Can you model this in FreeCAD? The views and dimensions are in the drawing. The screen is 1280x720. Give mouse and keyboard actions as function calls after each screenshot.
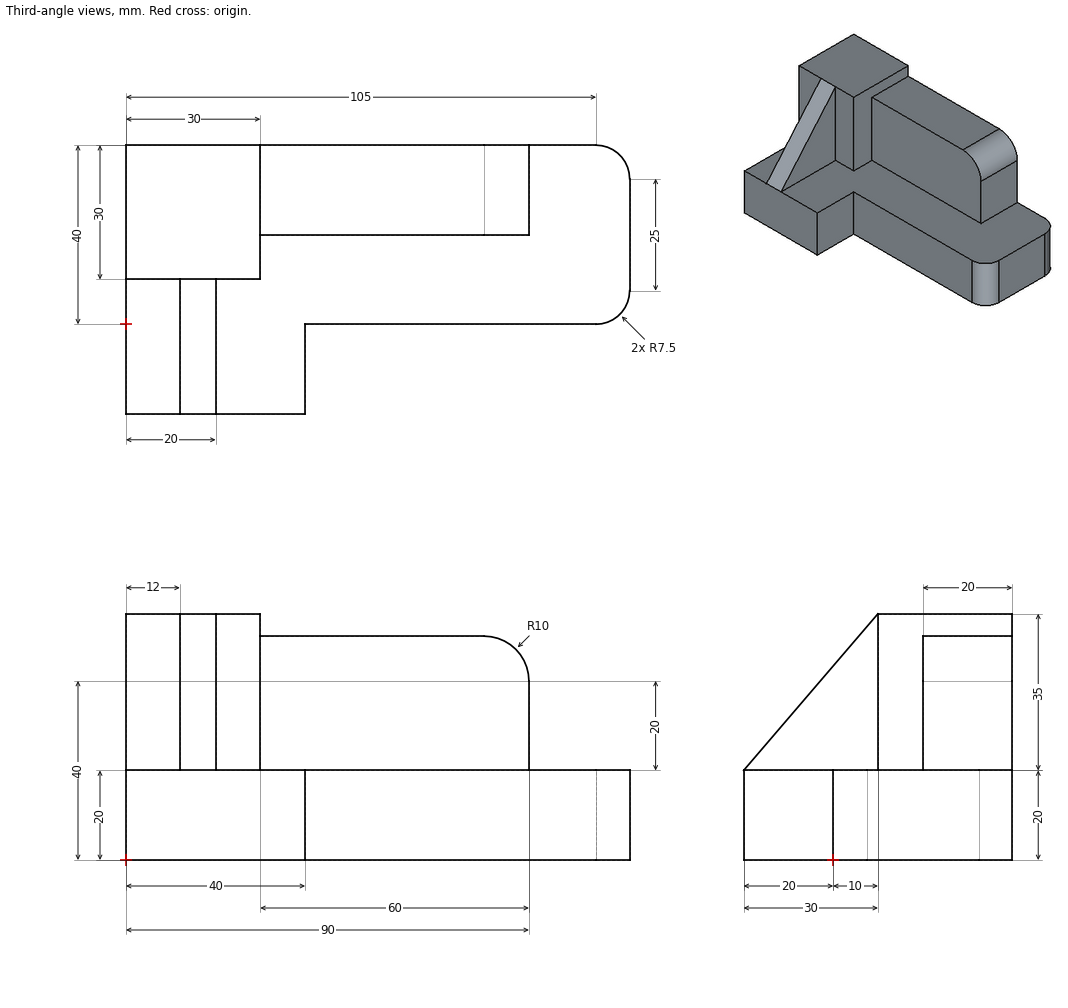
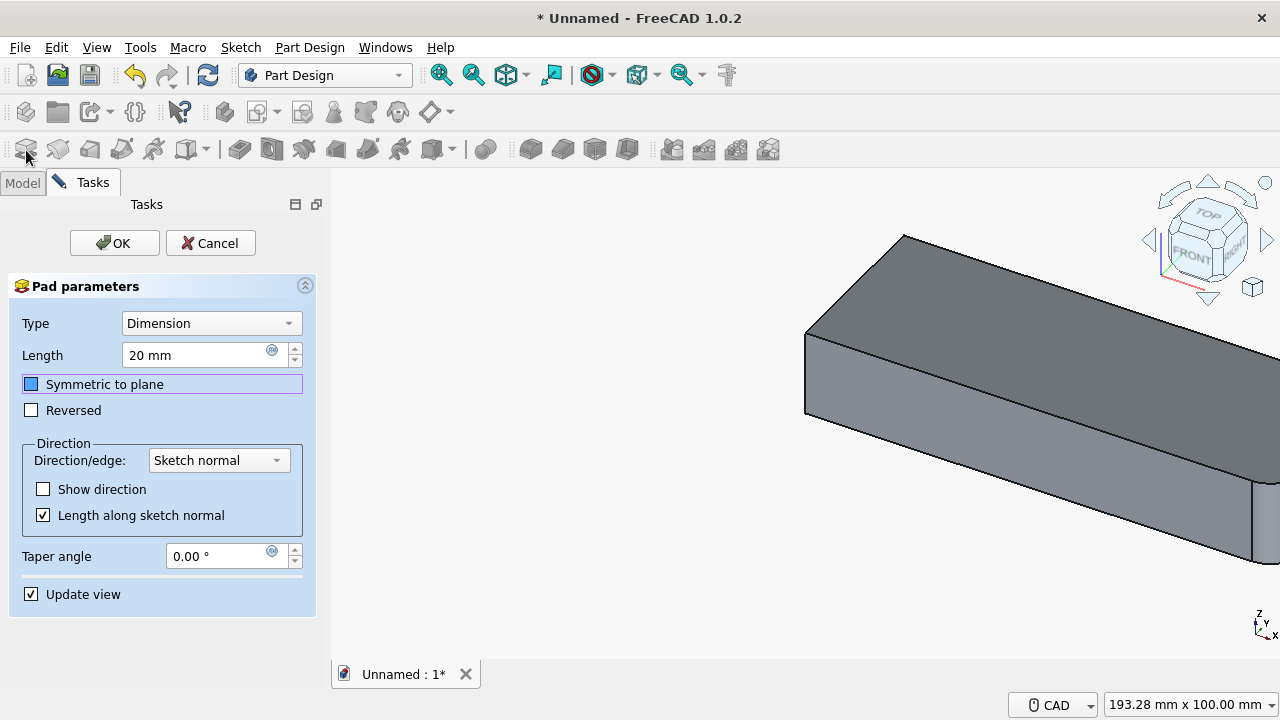
click(115, 243)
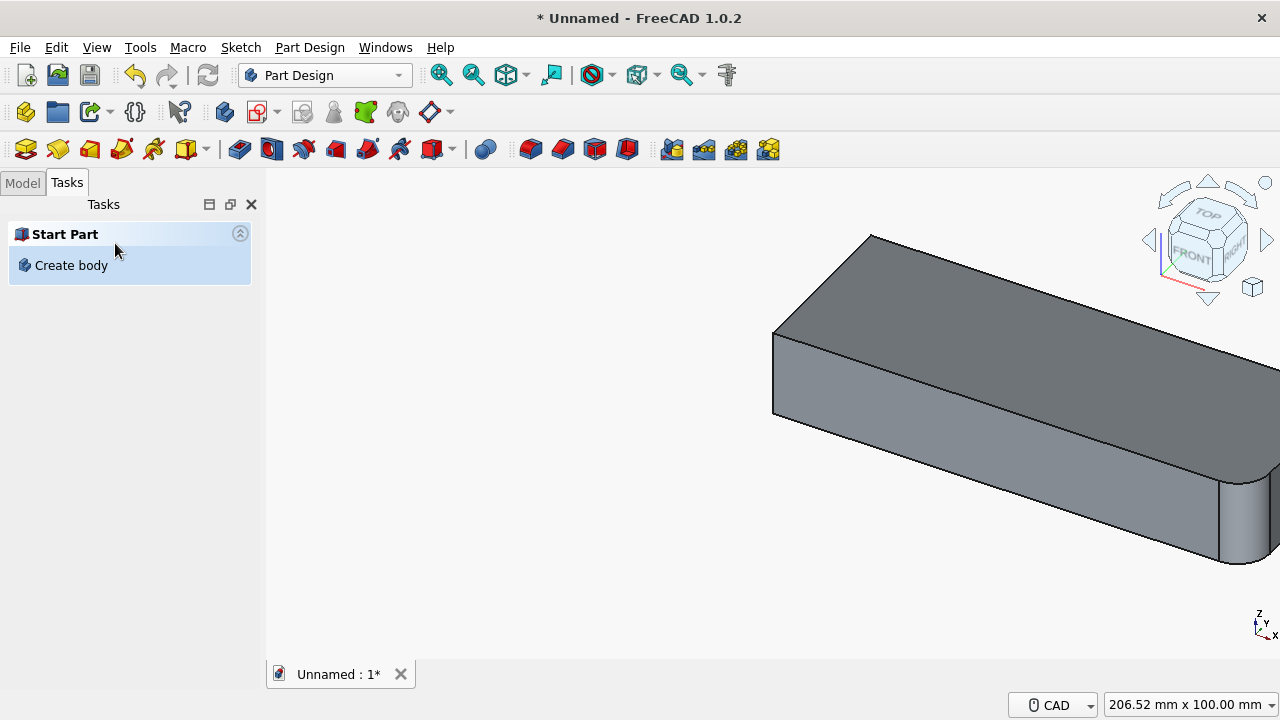
click(442, 76)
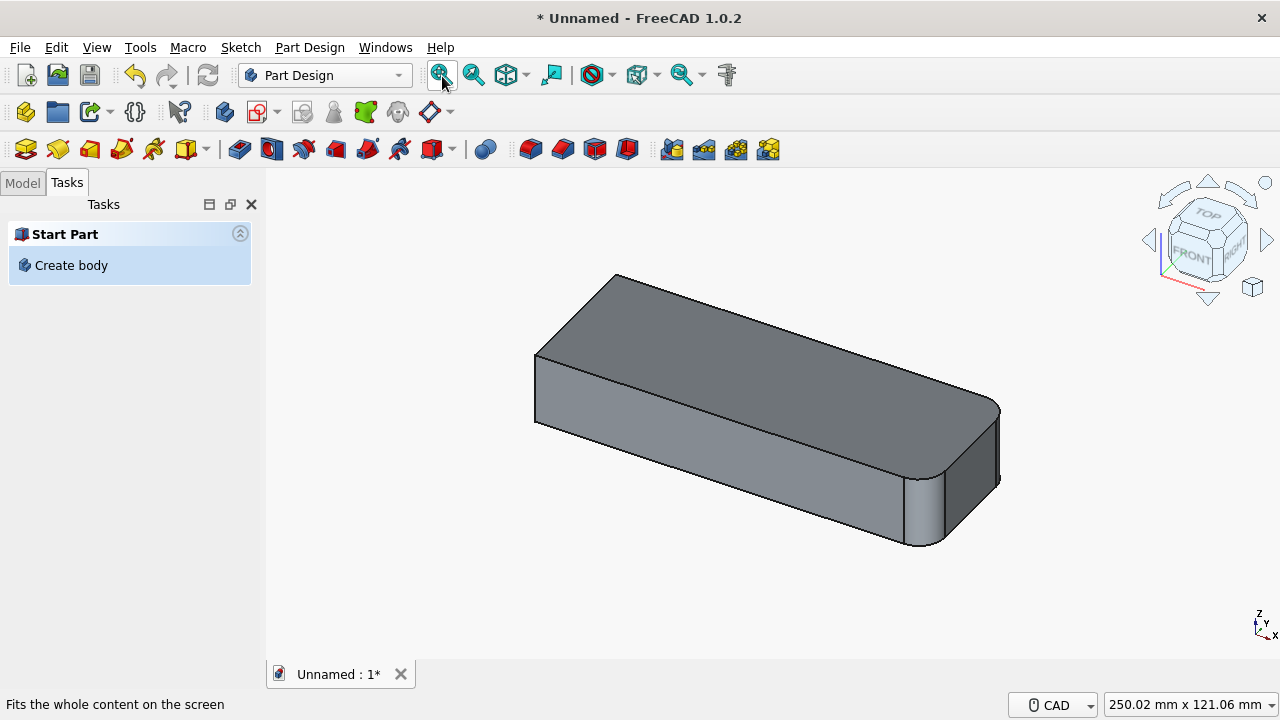
click(825, 483)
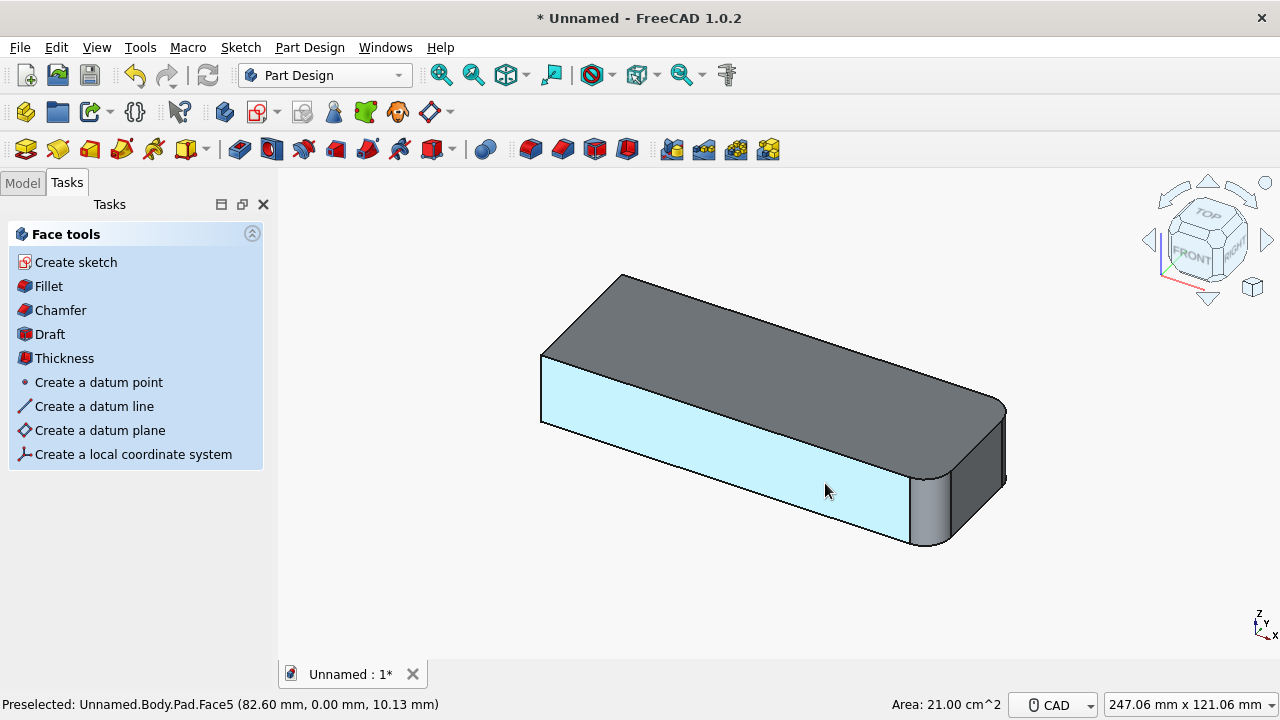
click(258, 112)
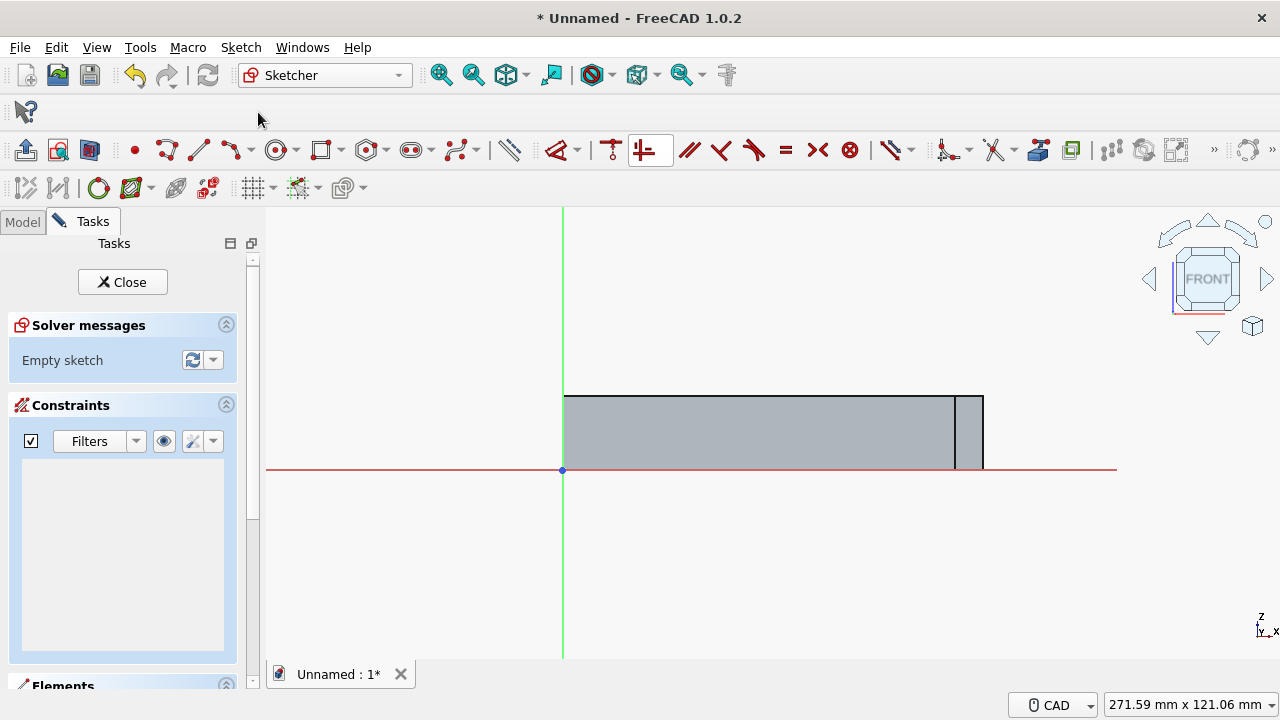
scroll(616, 433, up, 7)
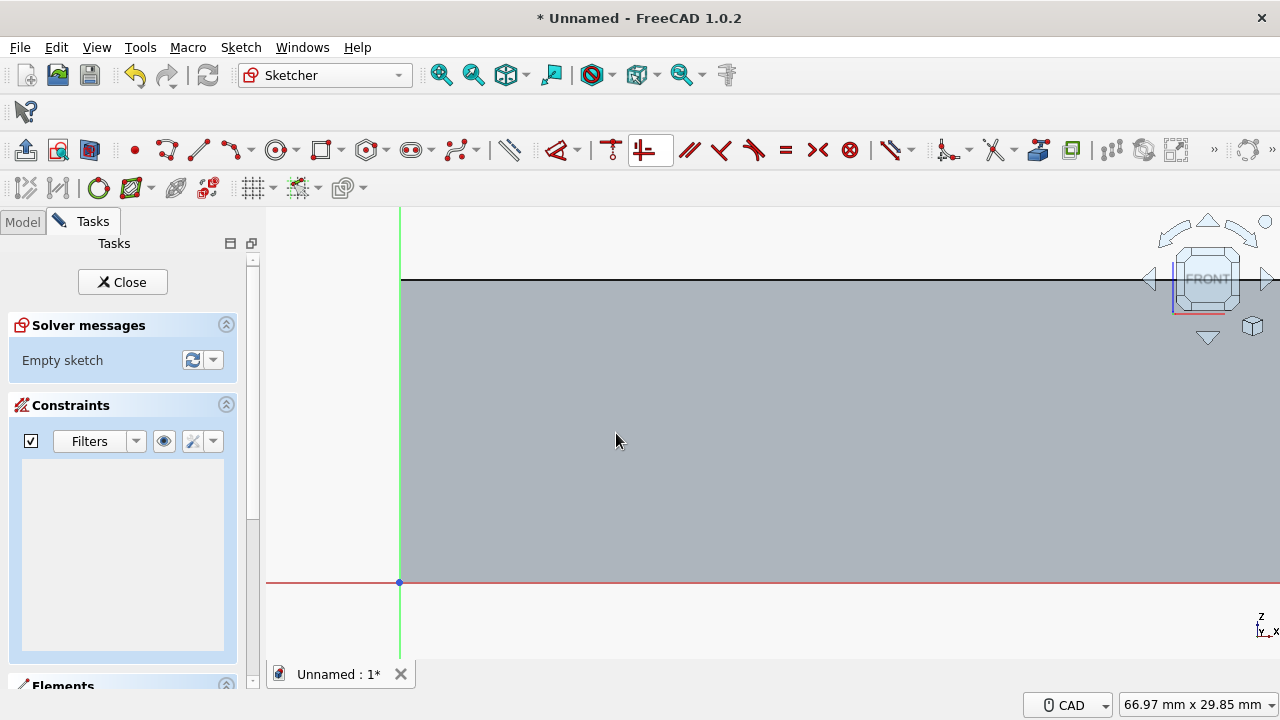
key(g)
key(r)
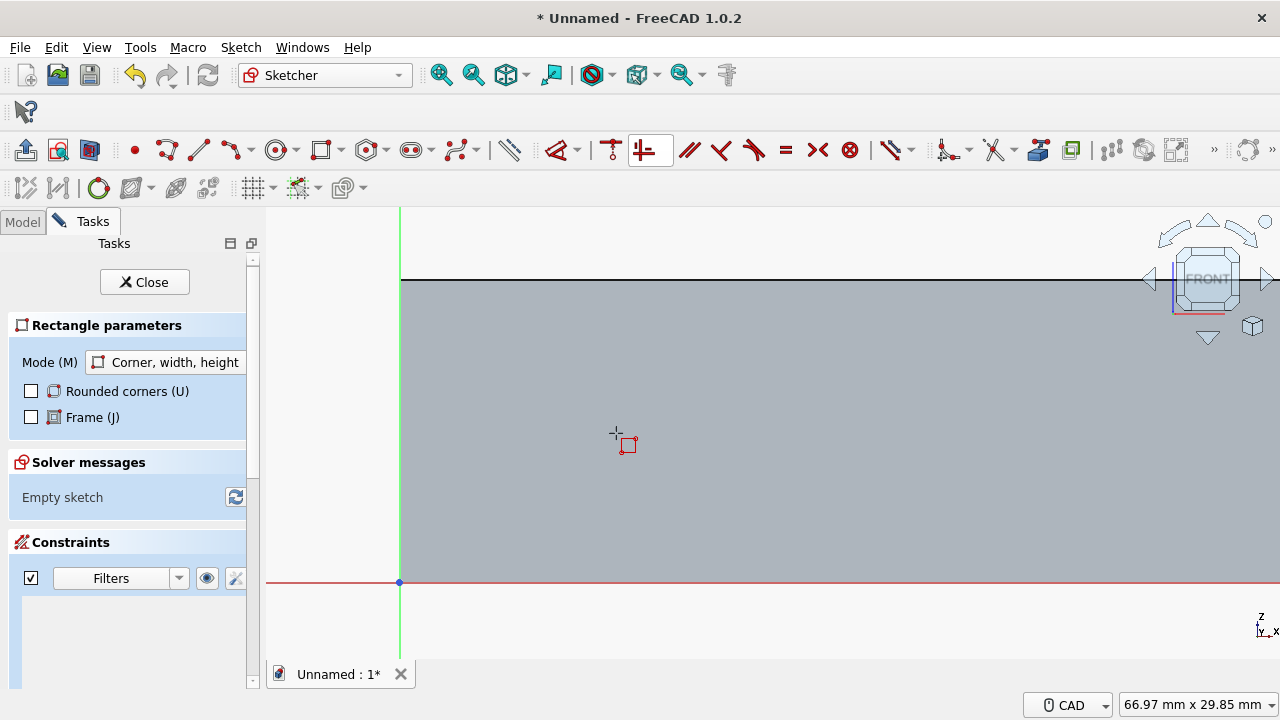
click(400, 583)
move(1006, 280)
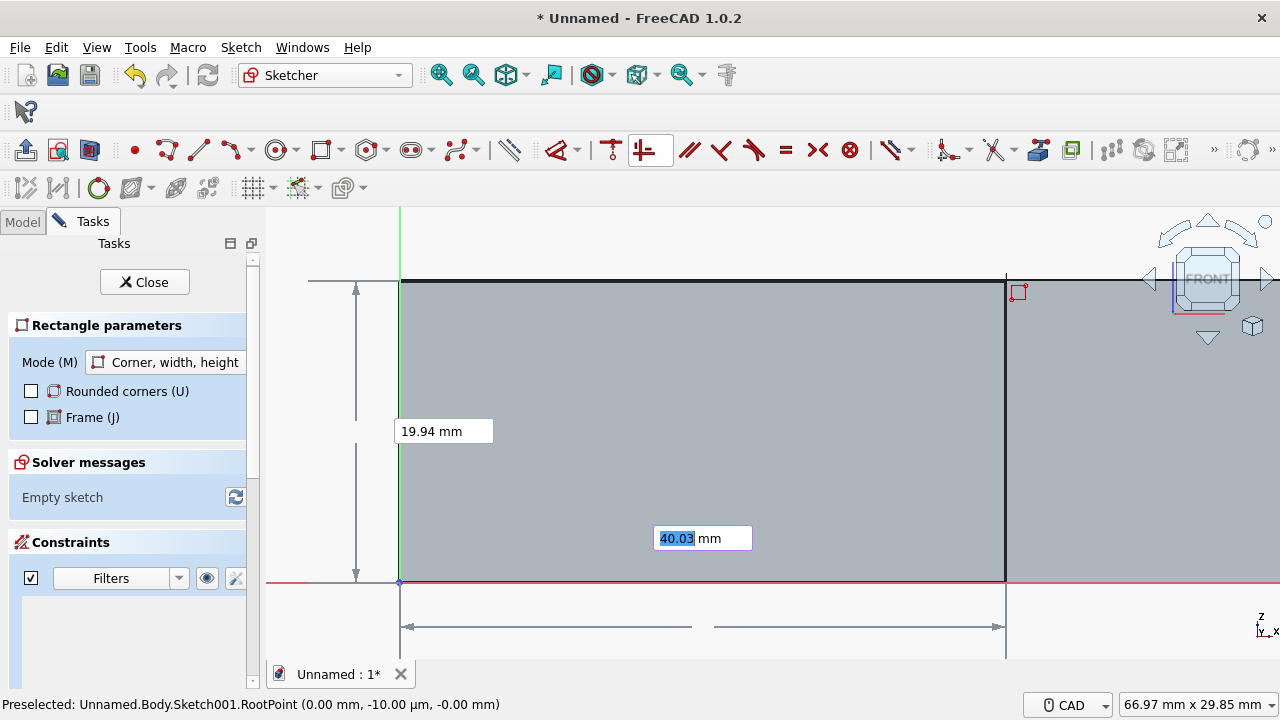
text(40)
key(Tab)
text(20)
key(Return)
key(Escape)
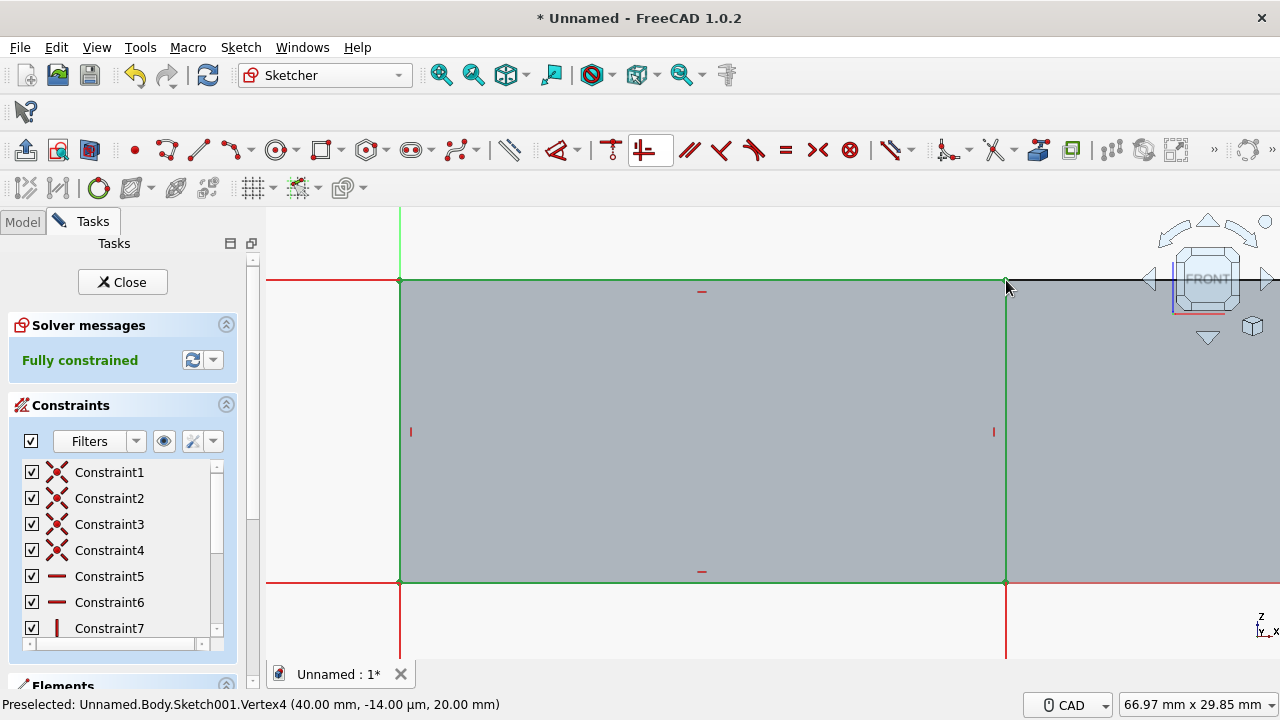
click(123, 282)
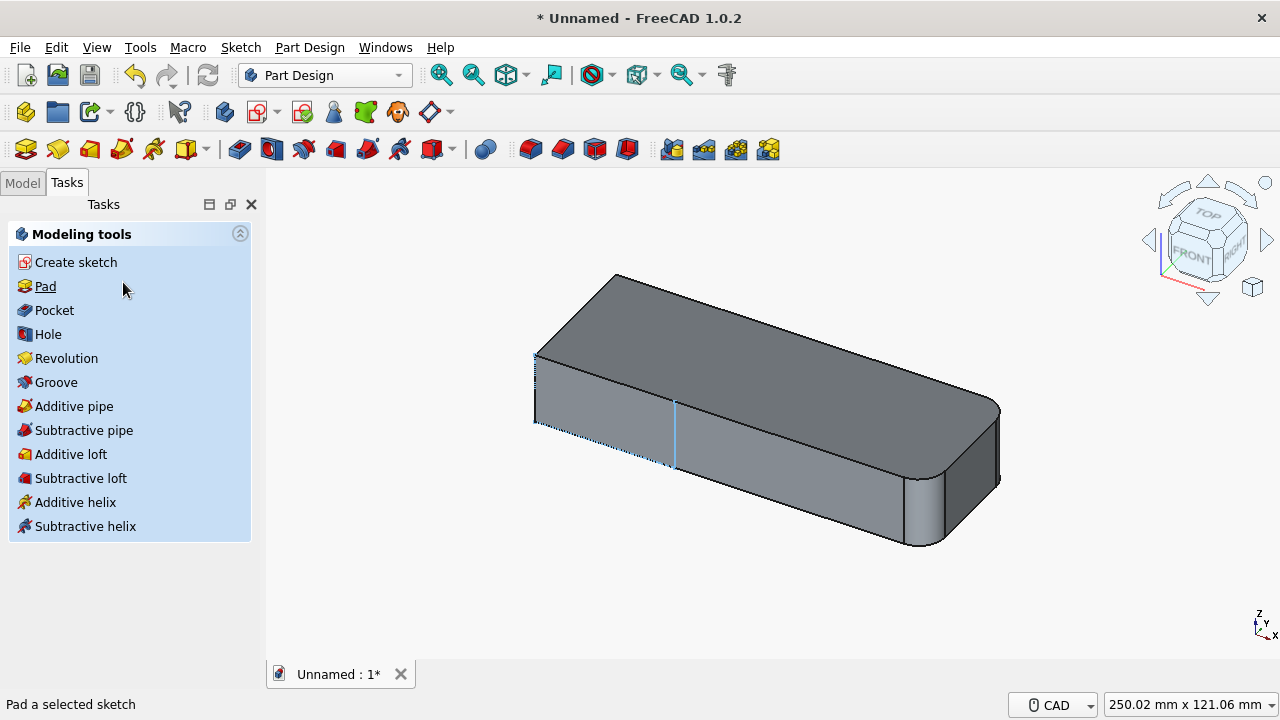
click(26, 150)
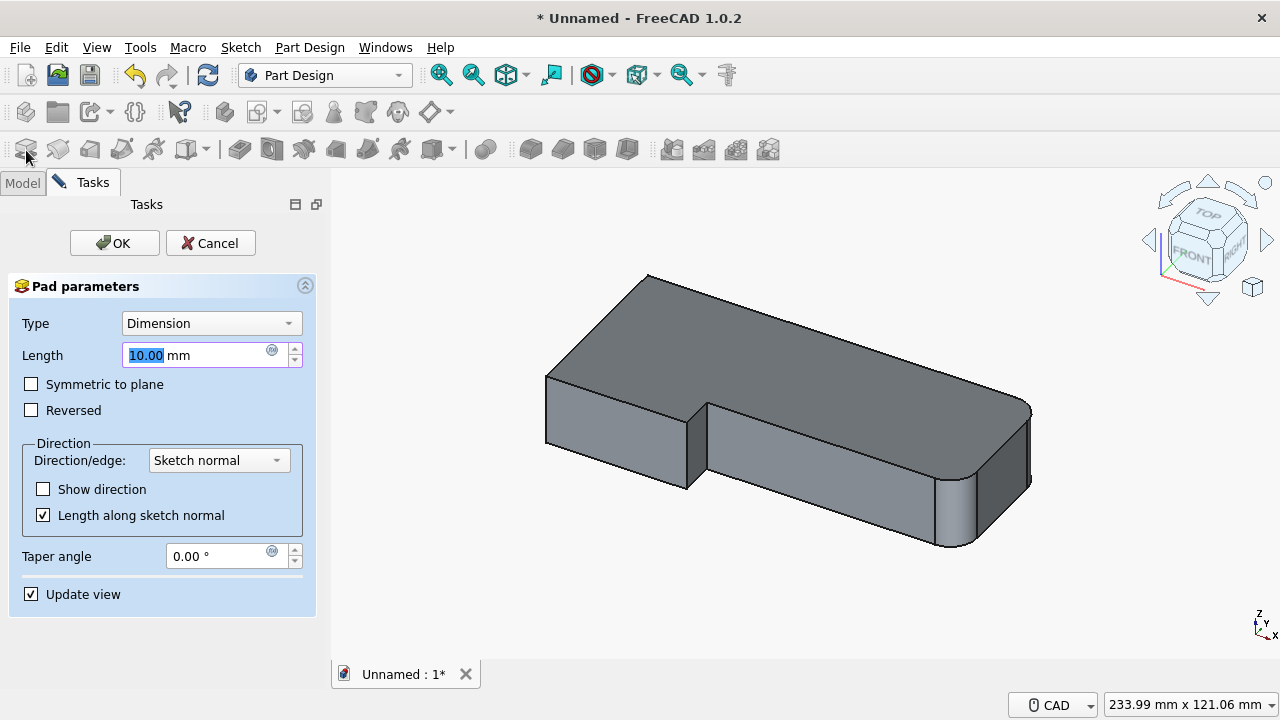
text(20)
key(Tab)